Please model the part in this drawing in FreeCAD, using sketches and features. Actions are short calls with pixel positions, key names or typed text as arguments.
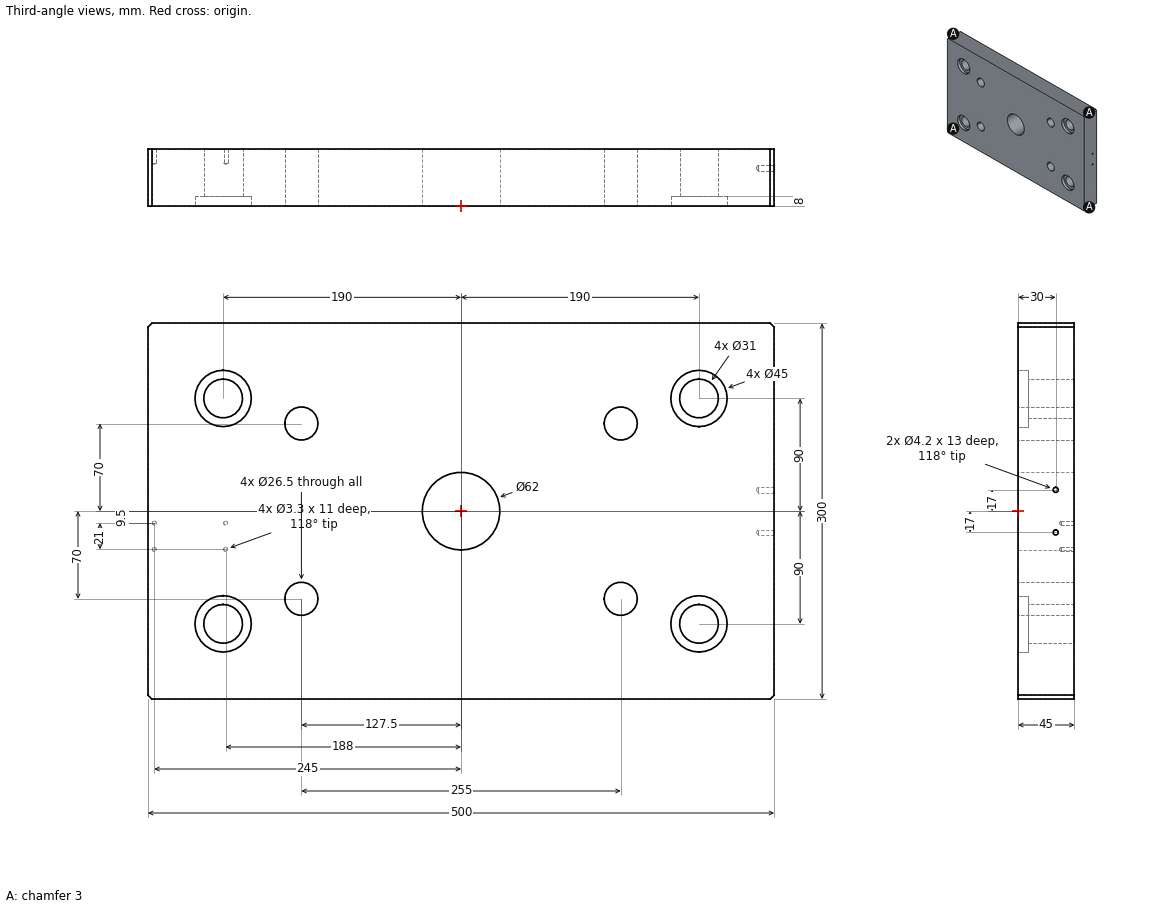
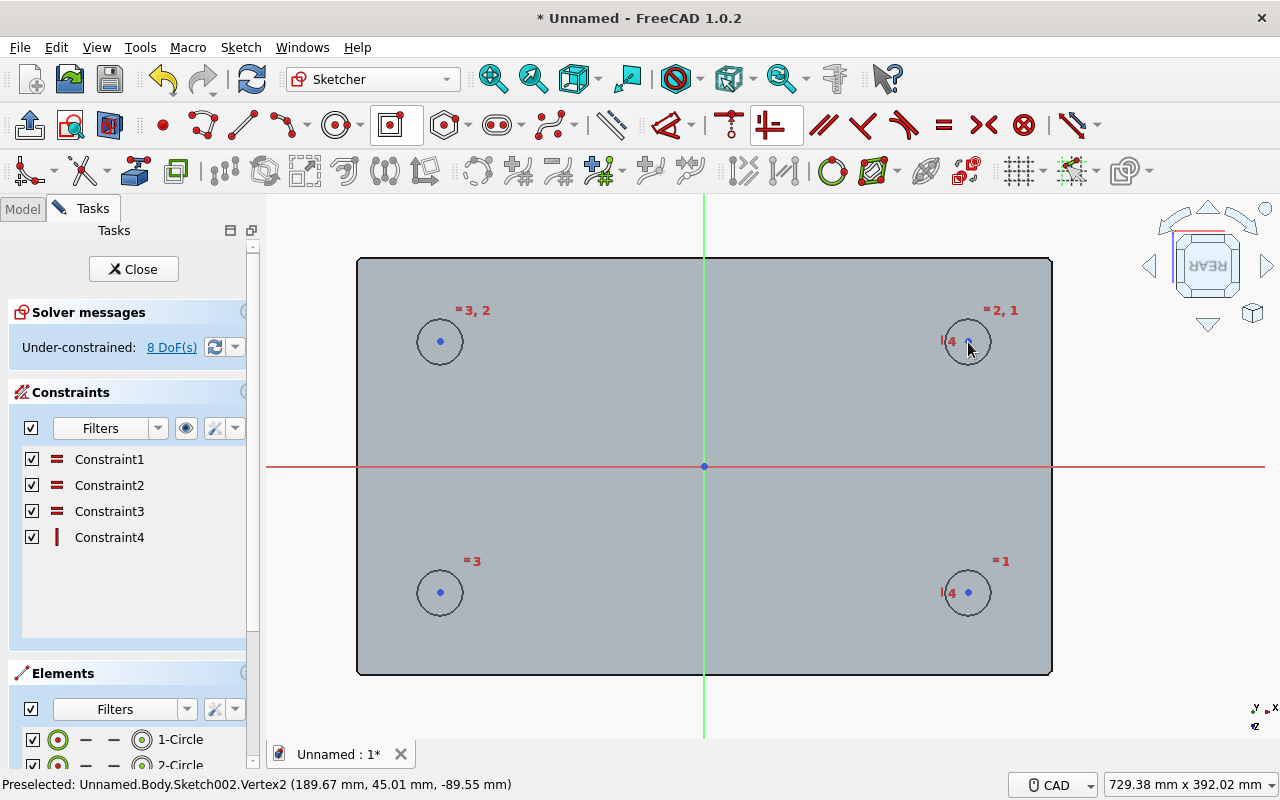
click(968, 342)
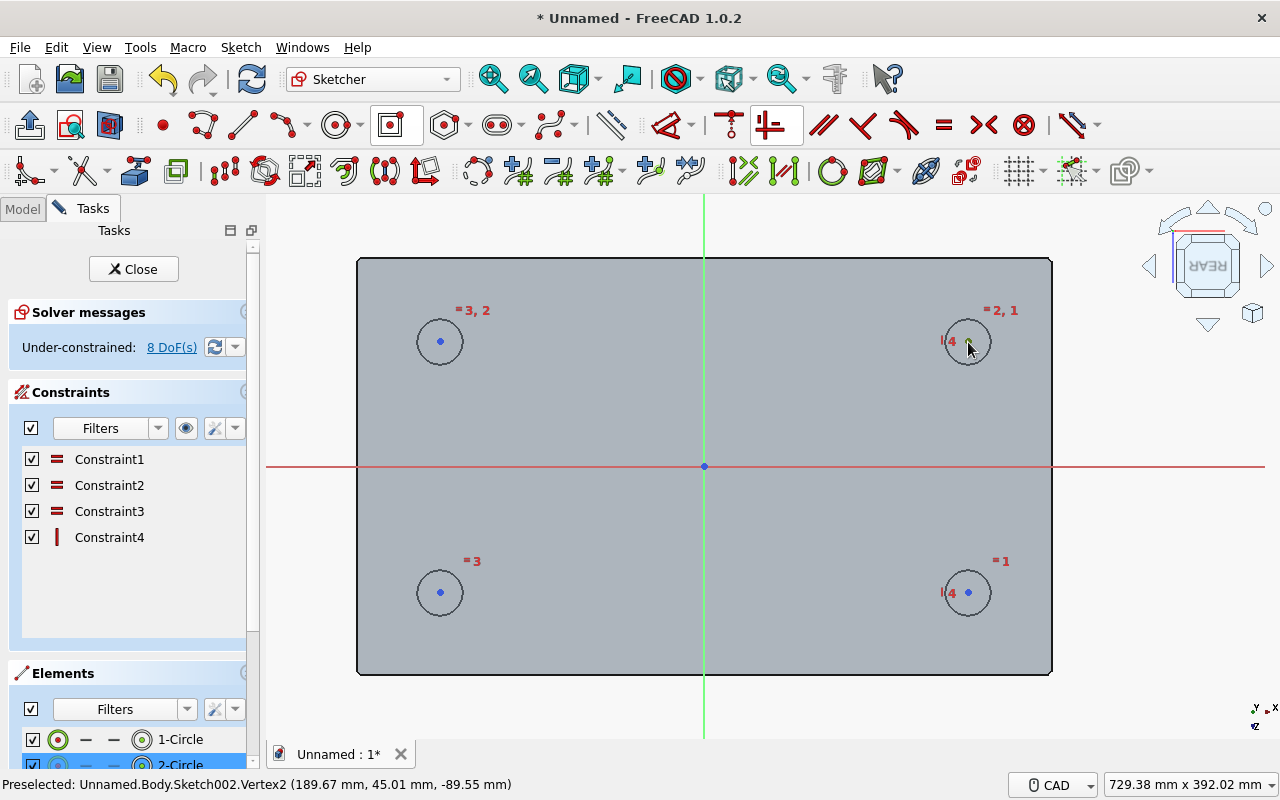
click(440, 342)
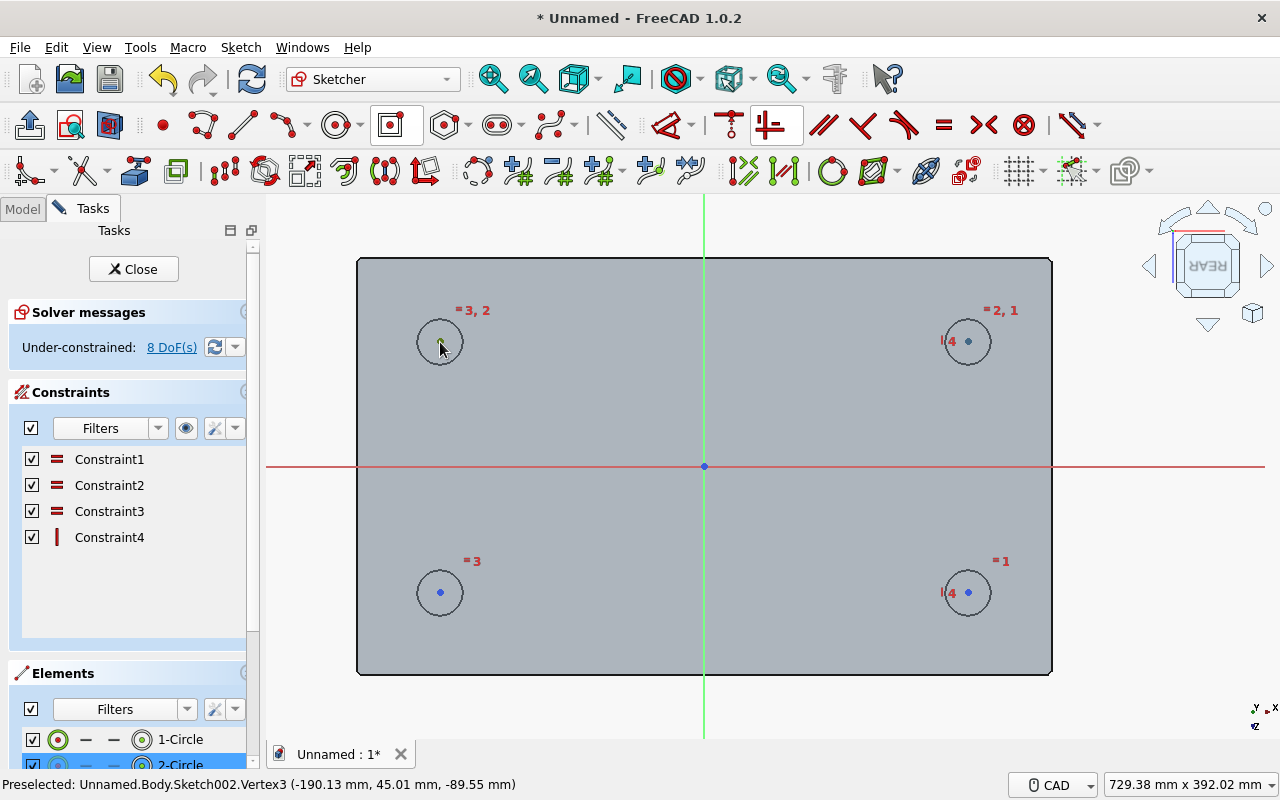
key(h)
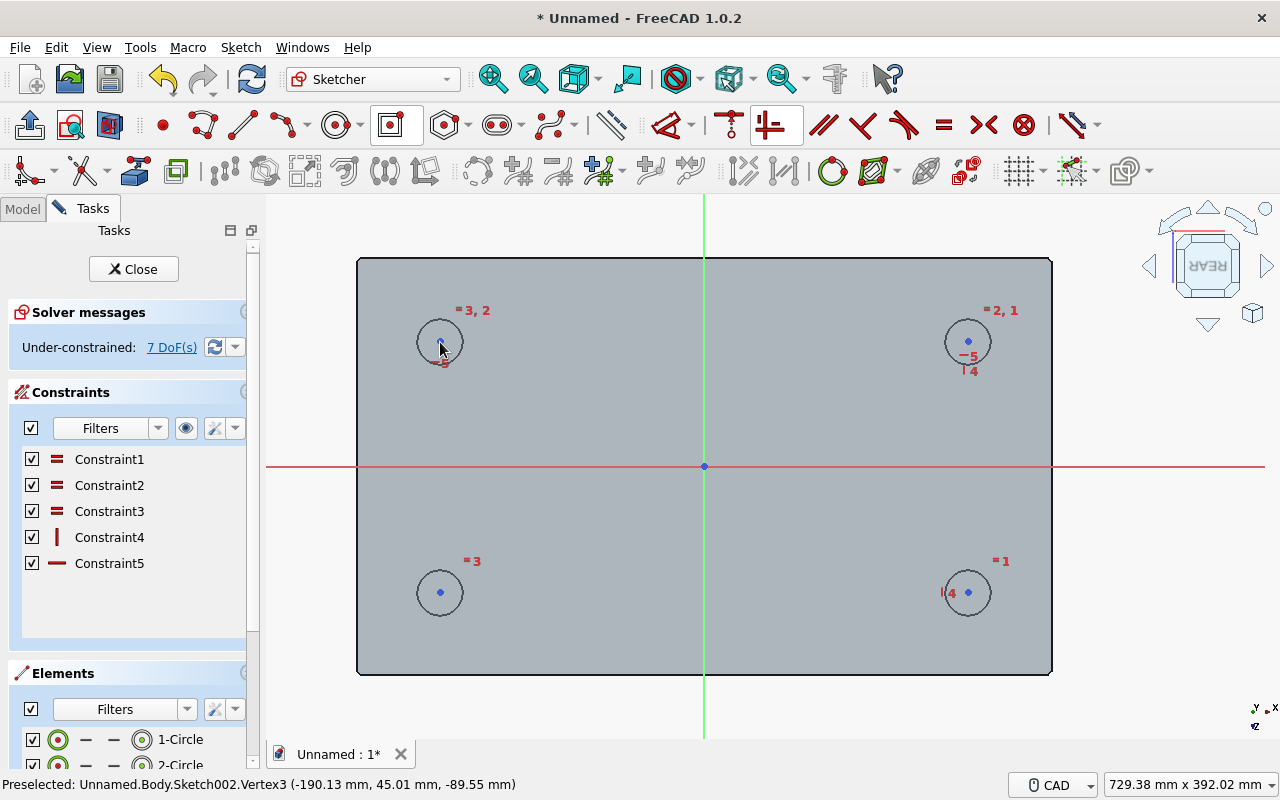
click(440, 342)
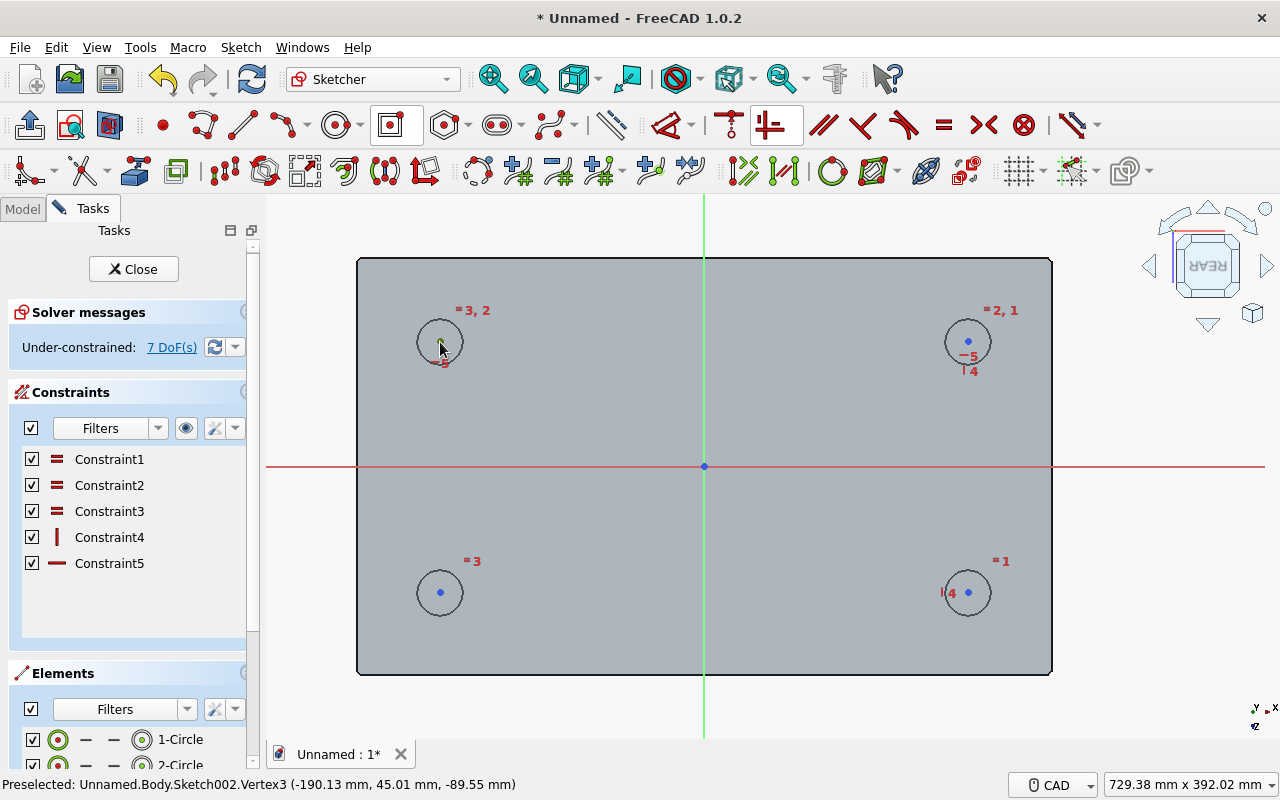
click(440, 593)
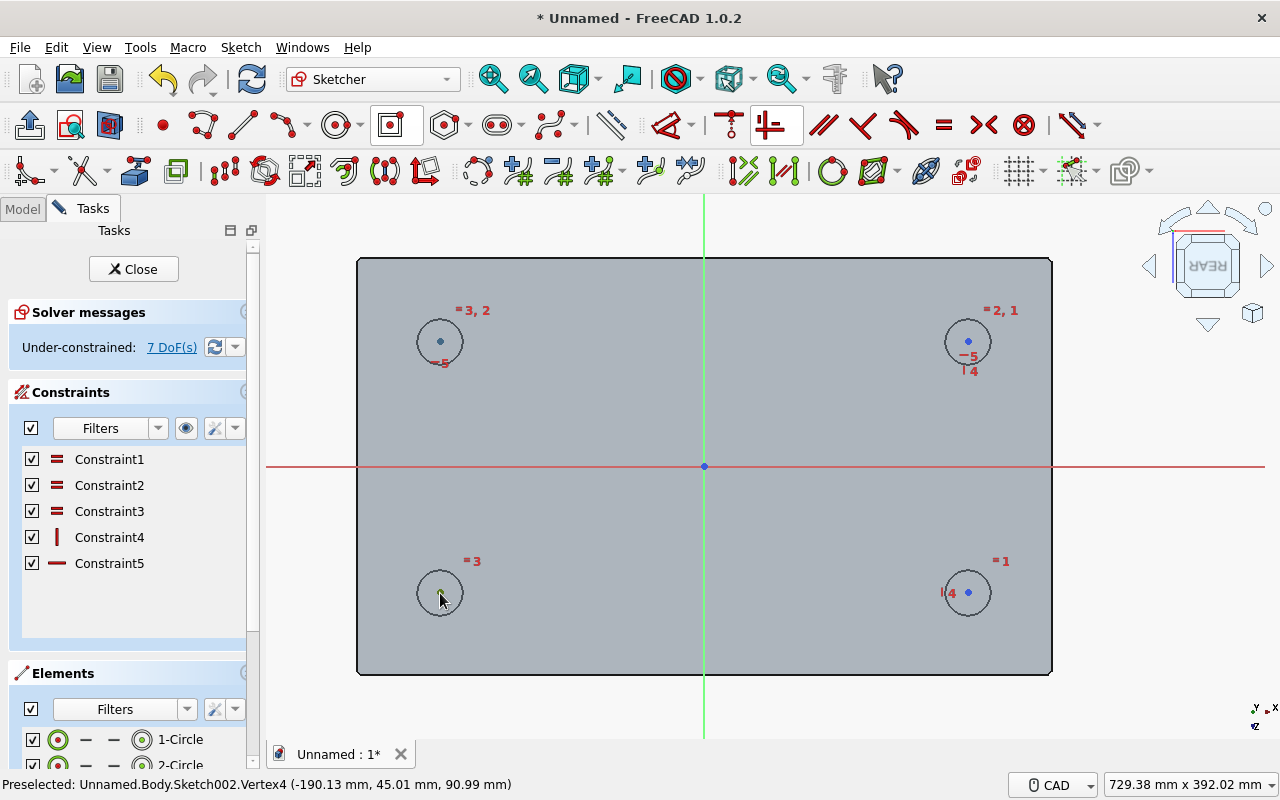
click(798, 126)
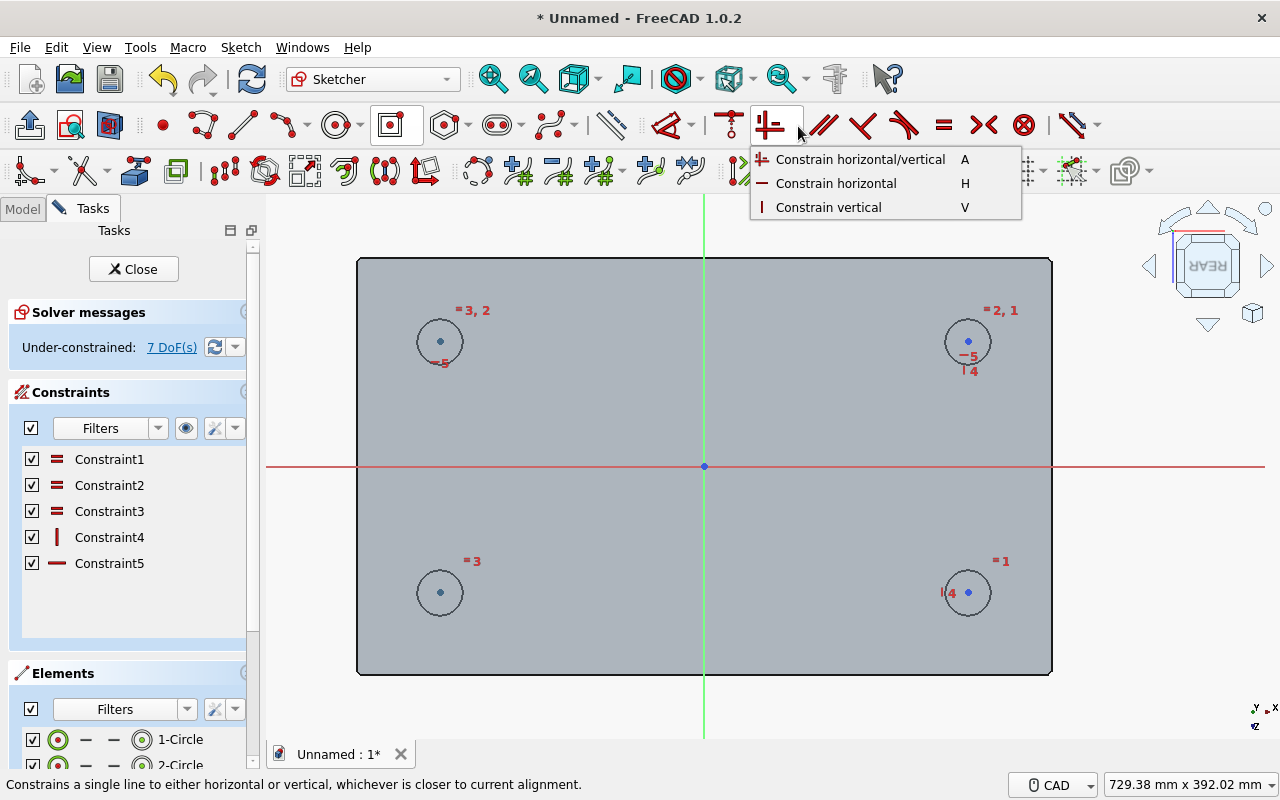
click(886, 207)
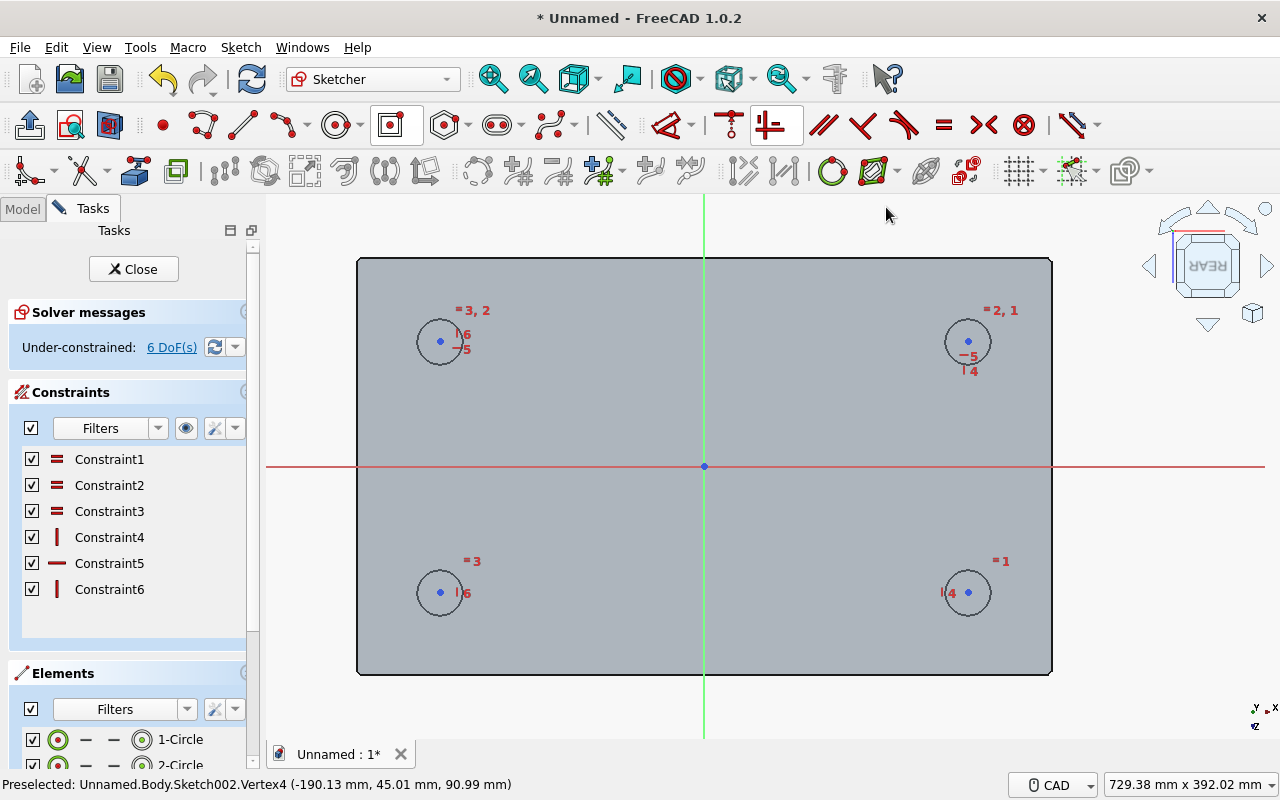
click(968, 593)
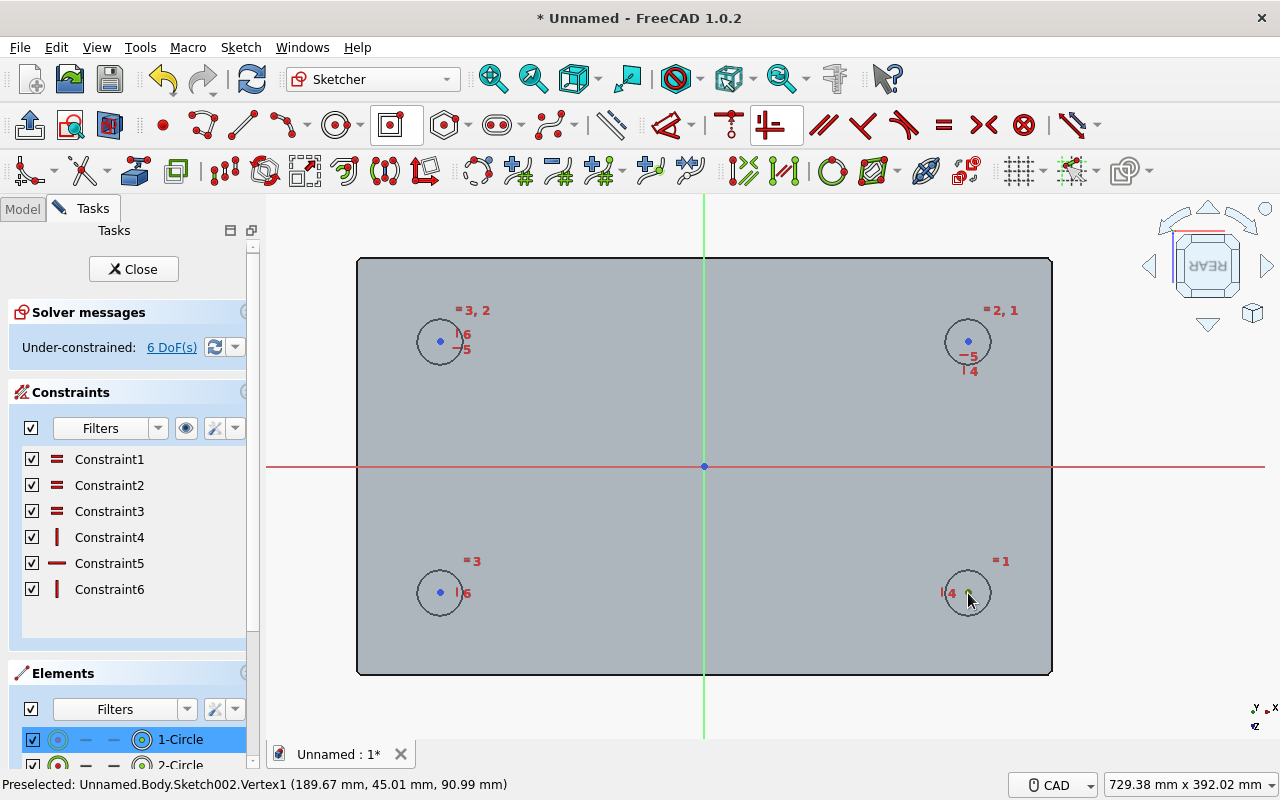
click(440, 593)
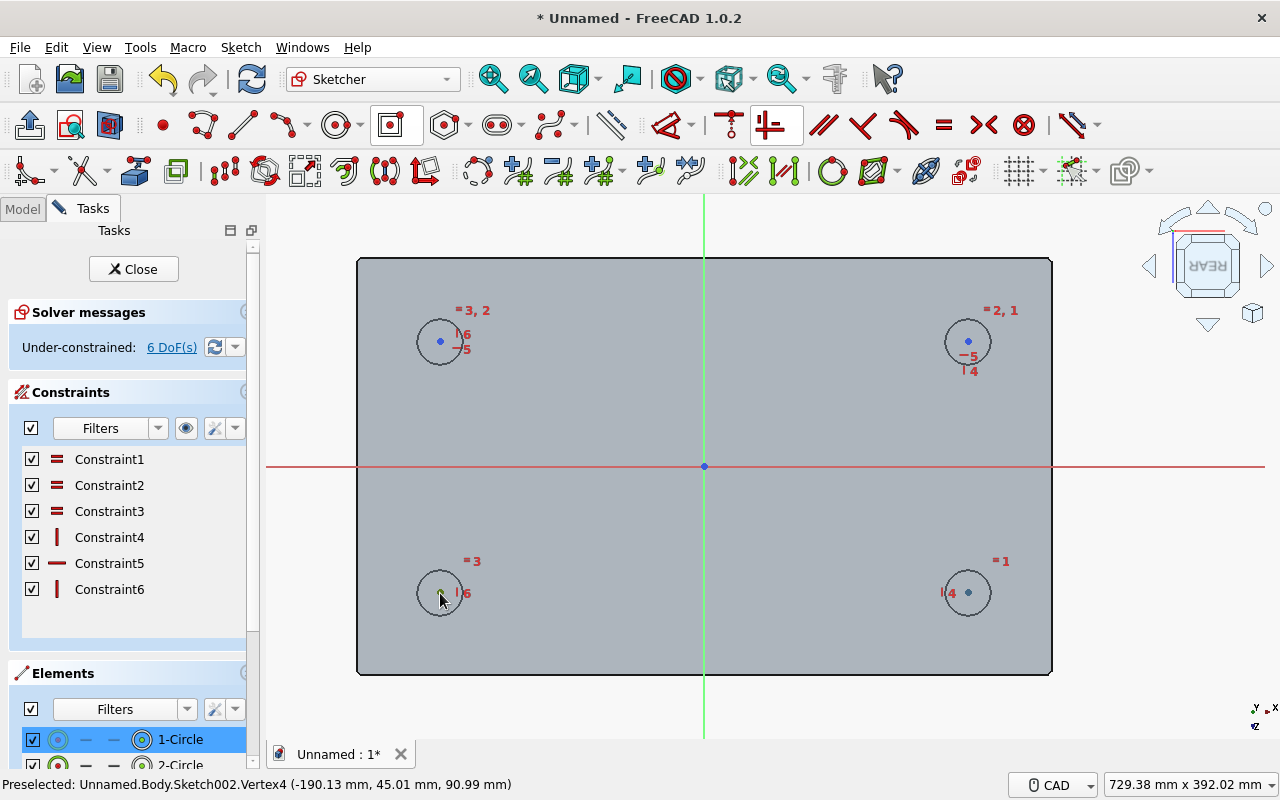
key(h)